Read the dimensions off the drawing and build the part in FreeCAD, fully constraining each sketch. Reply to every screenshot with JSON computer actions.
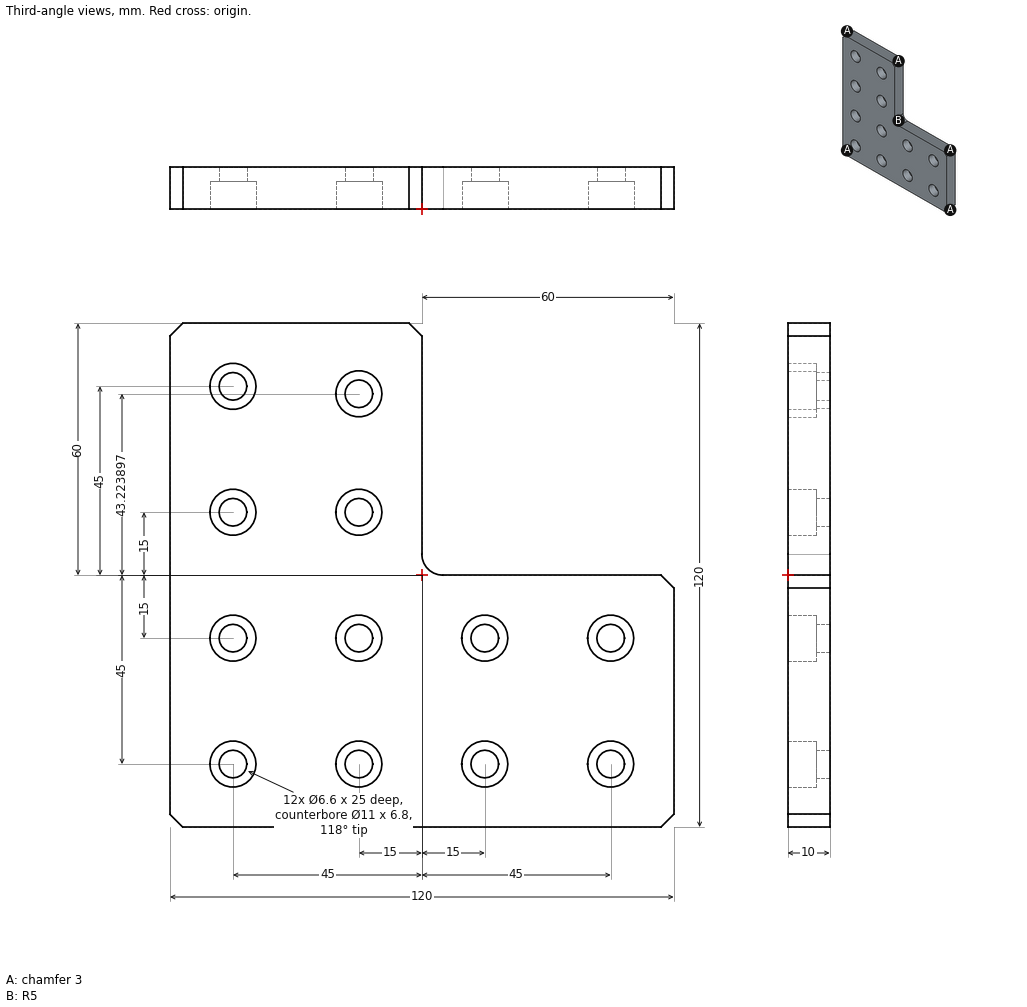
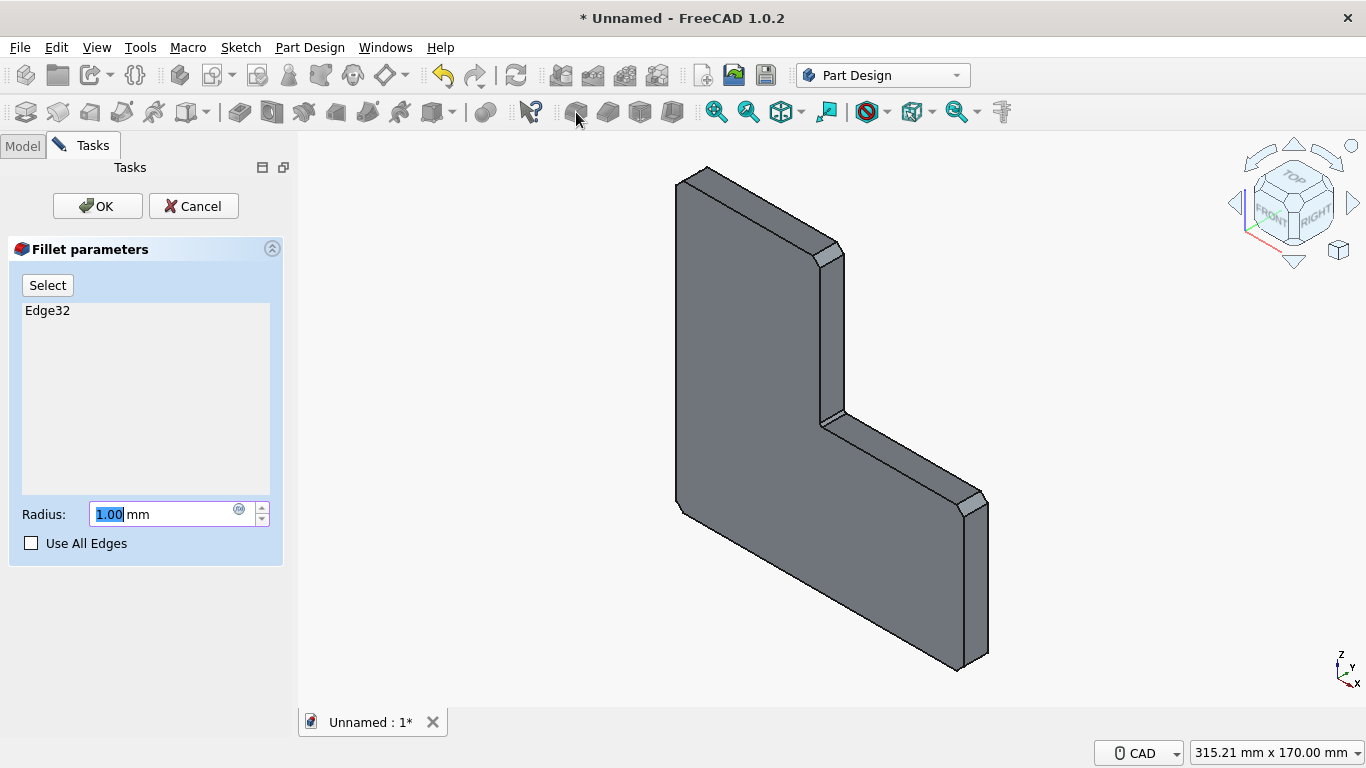
{"action": "type", "text": "5"}
{"action": "key", "text": "Tab"}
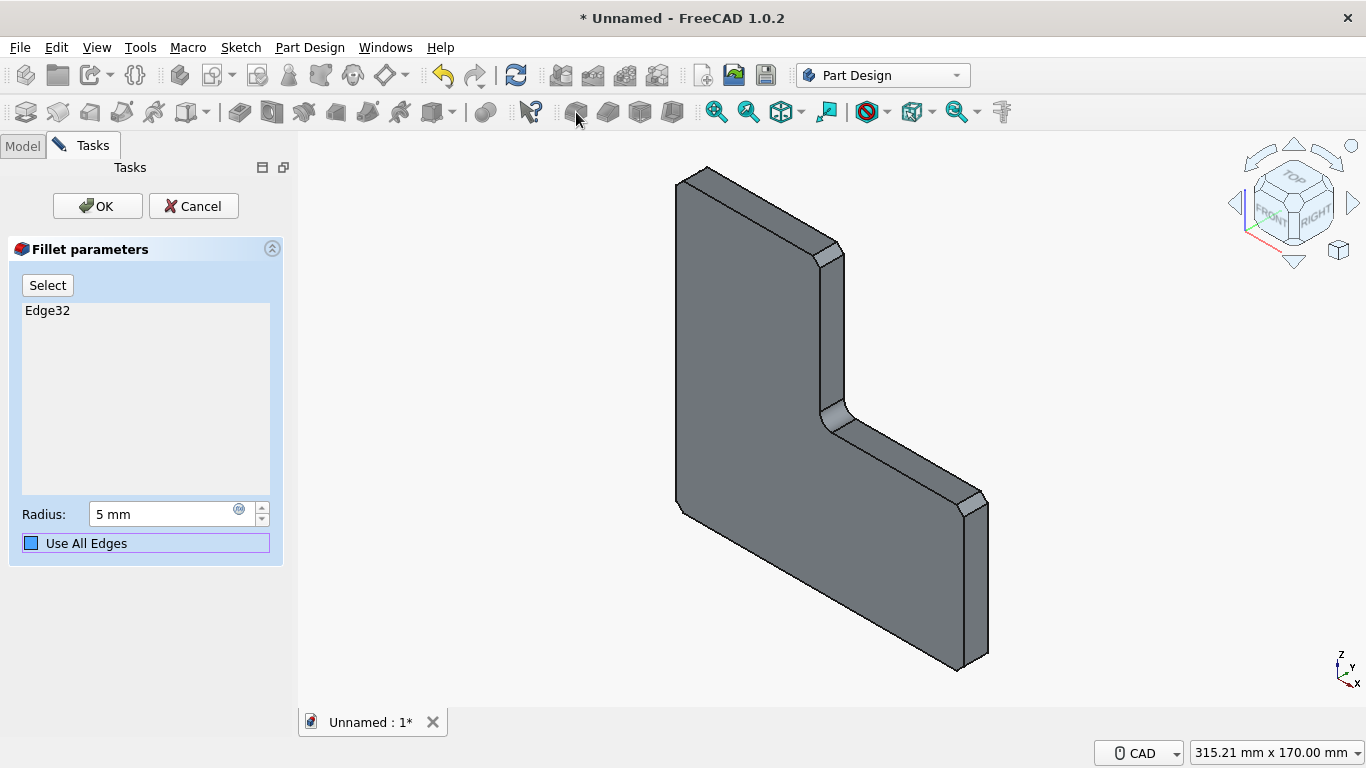
{"action": "left_click", "coordinate": [98, 206]}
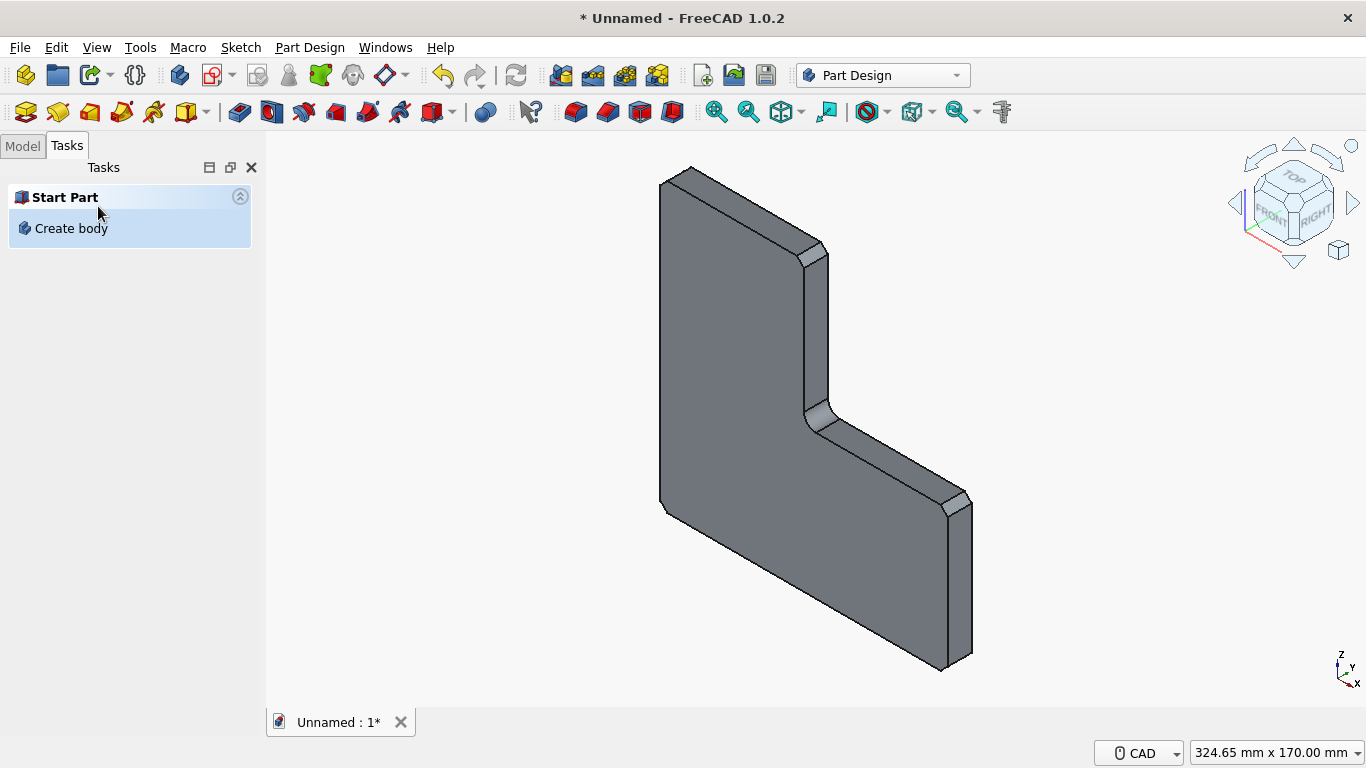
{"action": "left_click", "coordinate": [212, 76]}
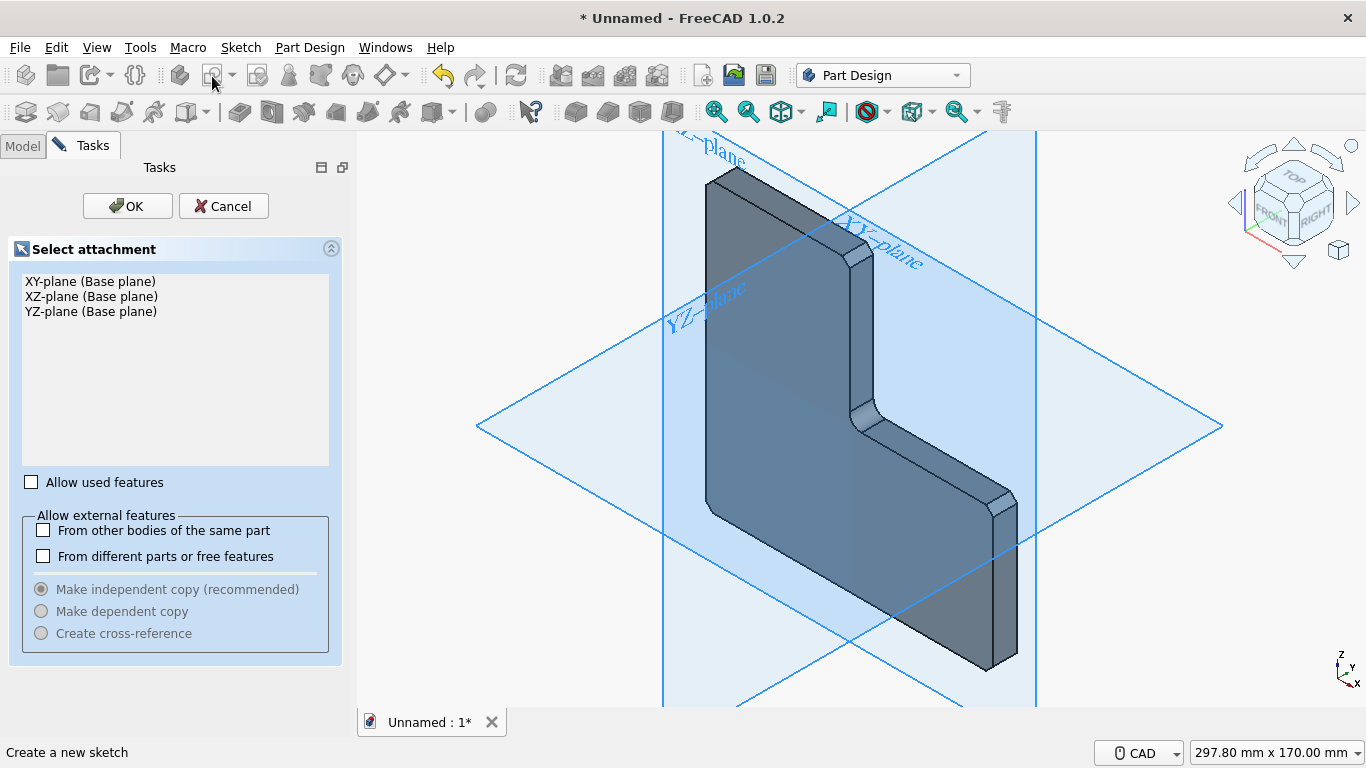
{"action": "left_click", "coordinate": [82, 296]}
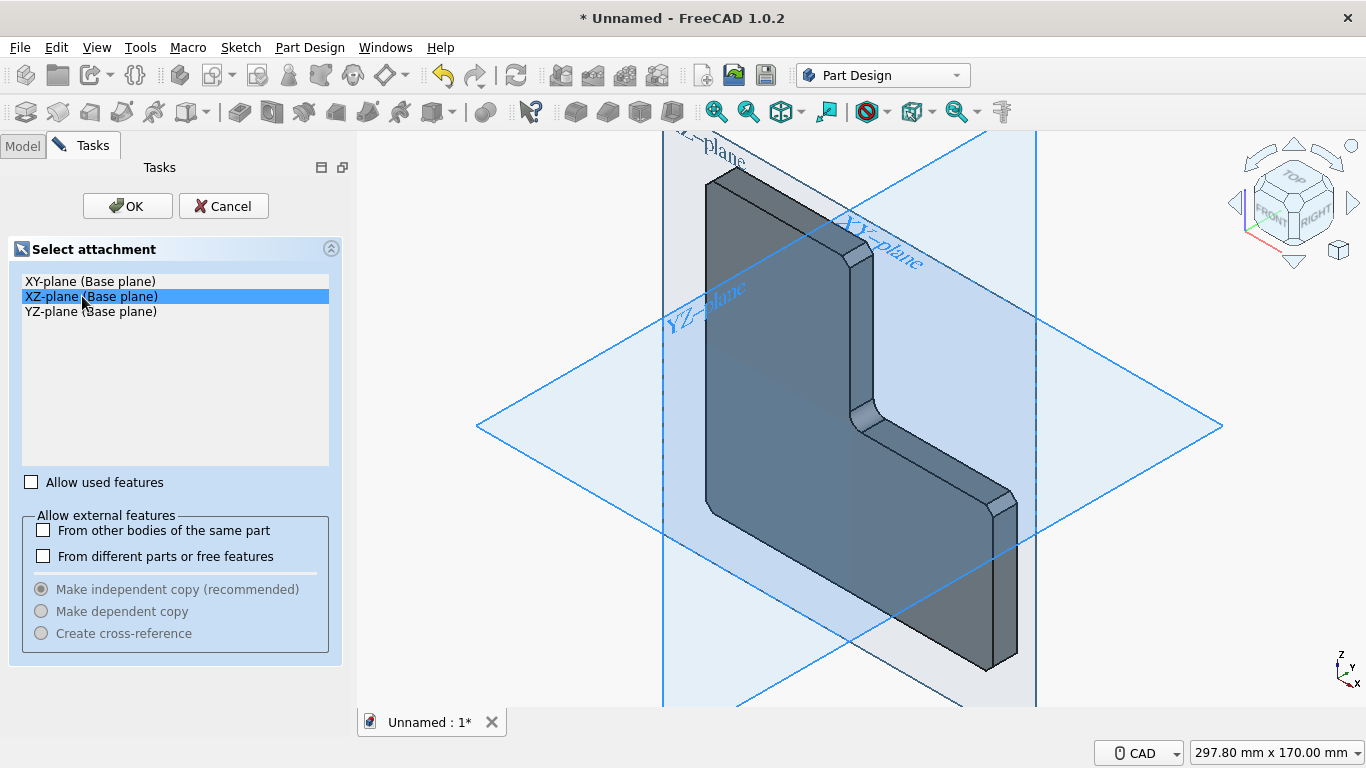
{"action": "left_click", "coordinate": [128, 206]}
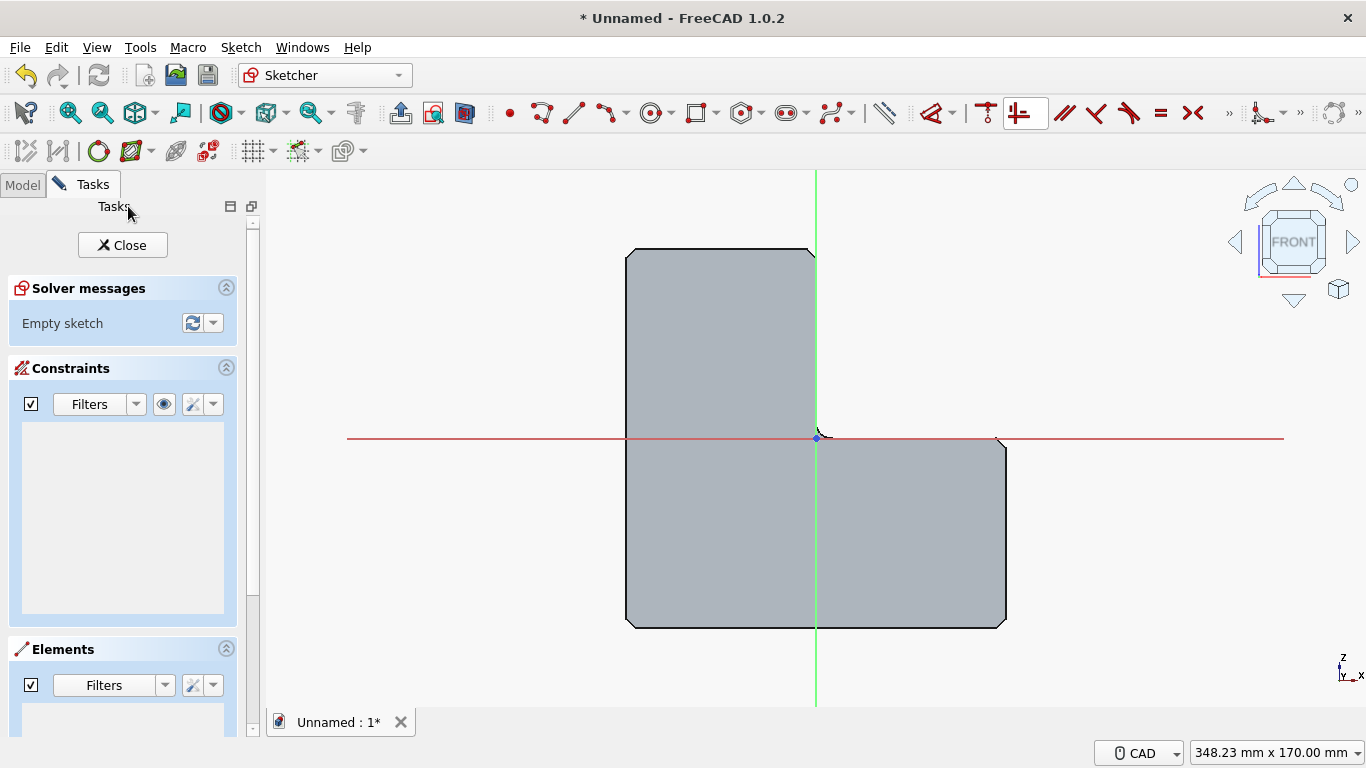
{"action": "left_click", "coordinate": [652, 114]}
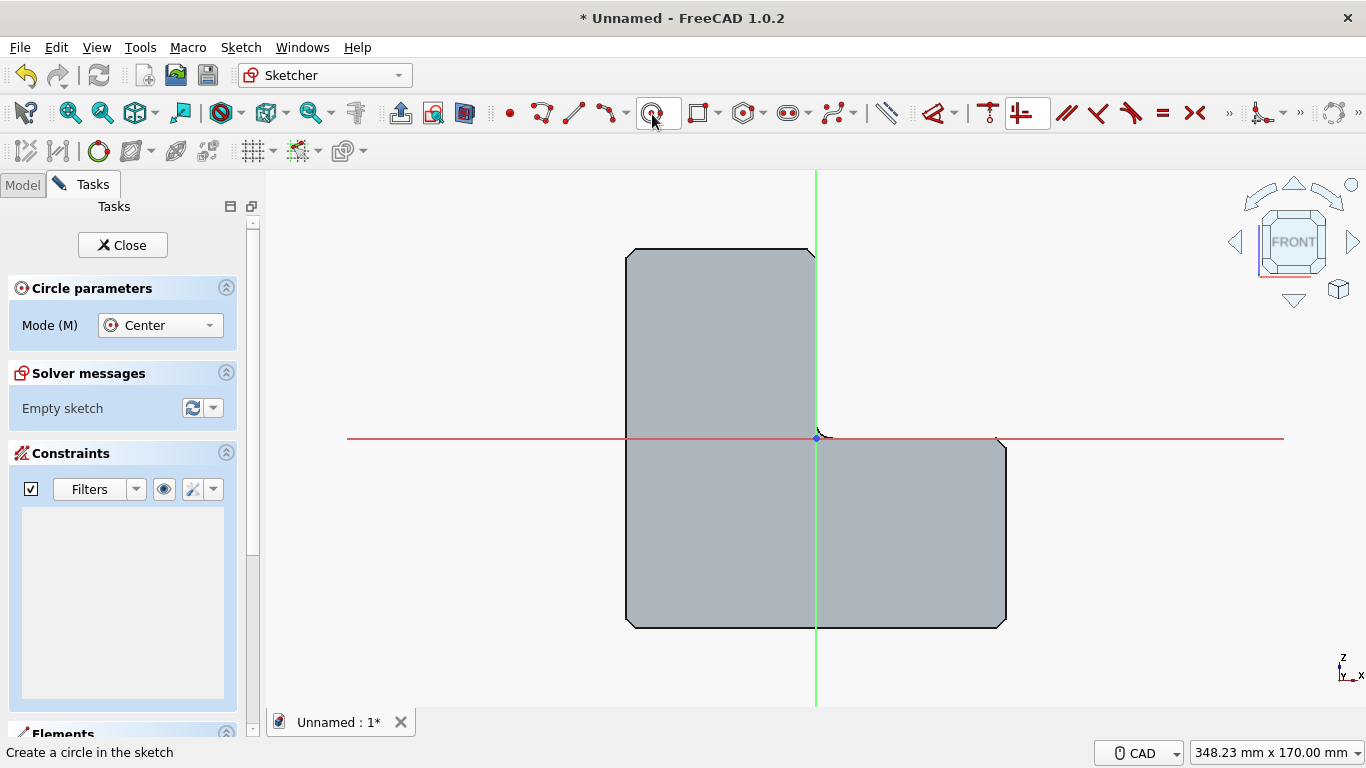
{"action": "scroll", "coordinate": [674, 581], "scroll_direction": "up", "scroll_amount": 4}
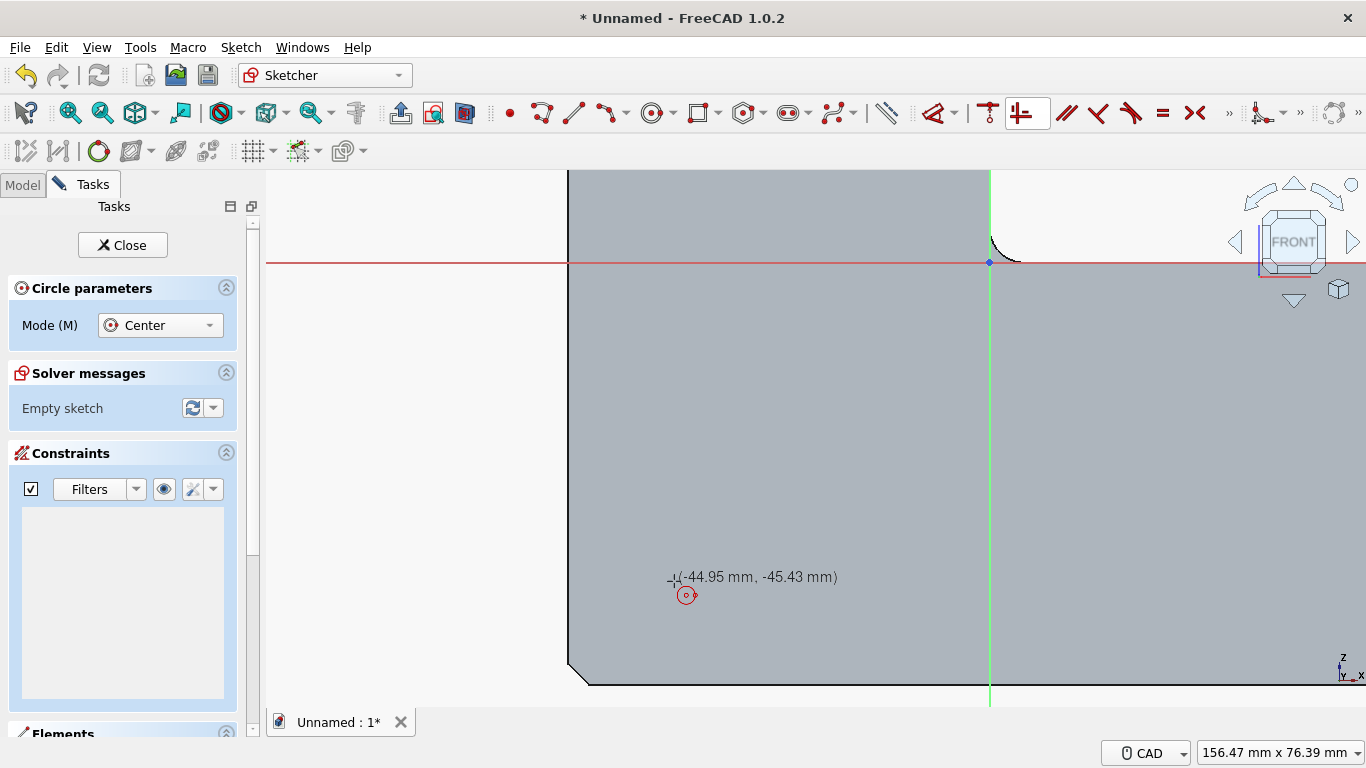
{"action": "left_click", "coordinate": [673, 579]}
{"action": "left_click", "coordinate": [690, 563]}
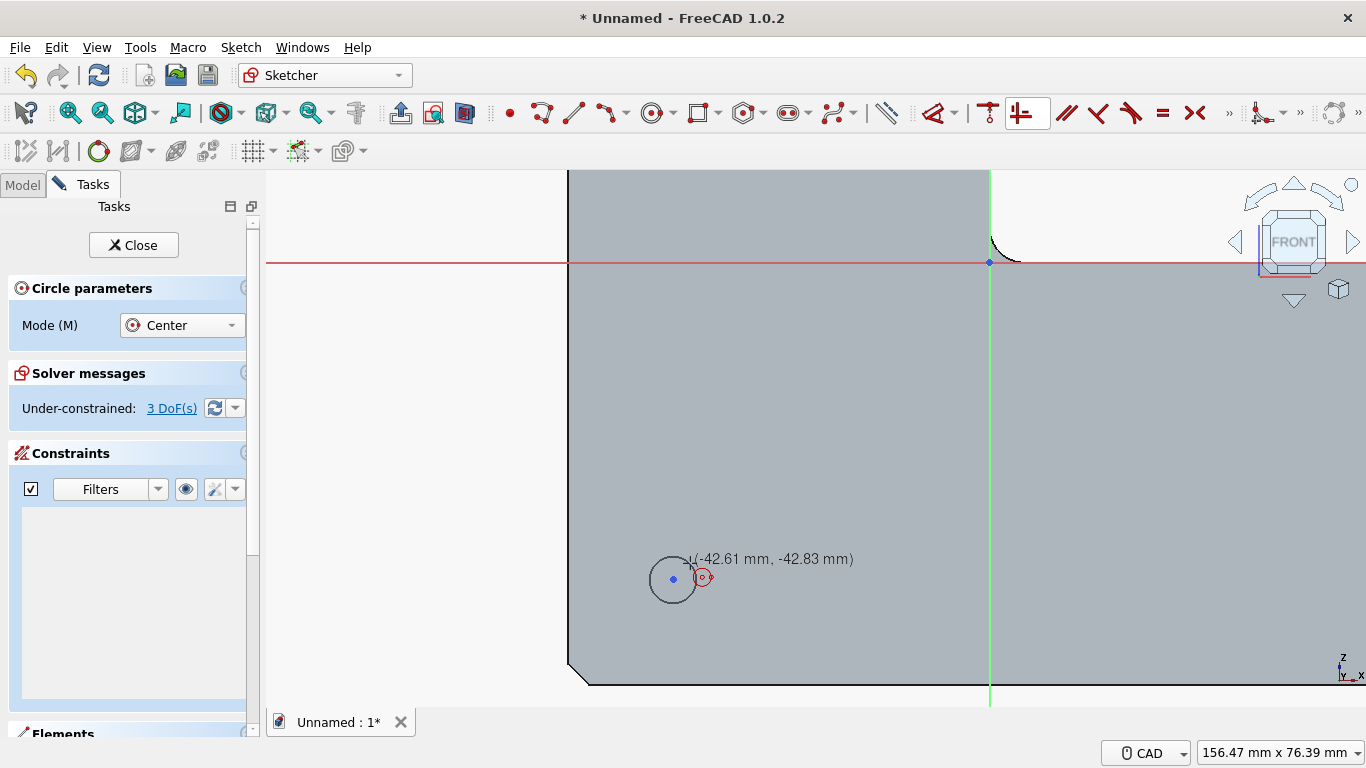
{"action": "left_click", "coordinate": [673, 368]}
{"action": "left_click", "coordinate": [690, 352]}